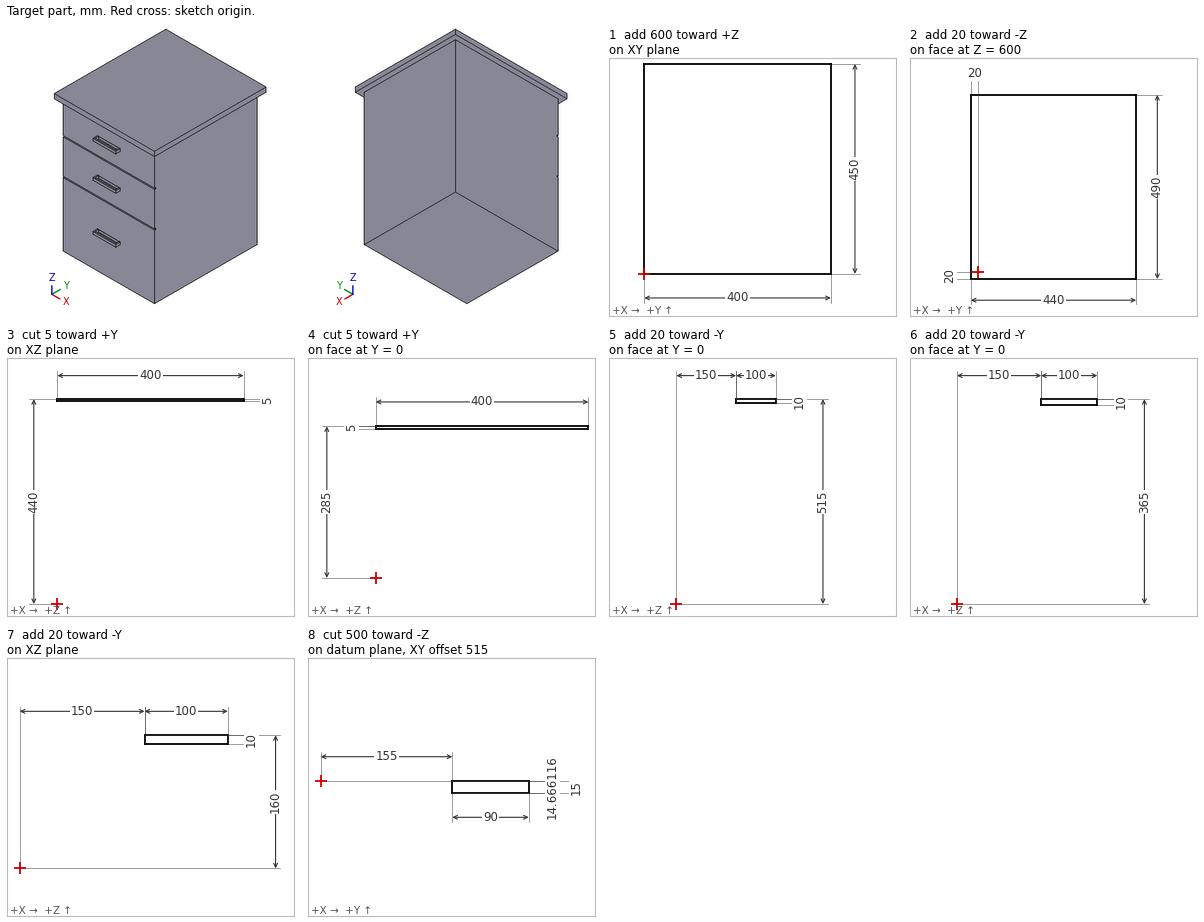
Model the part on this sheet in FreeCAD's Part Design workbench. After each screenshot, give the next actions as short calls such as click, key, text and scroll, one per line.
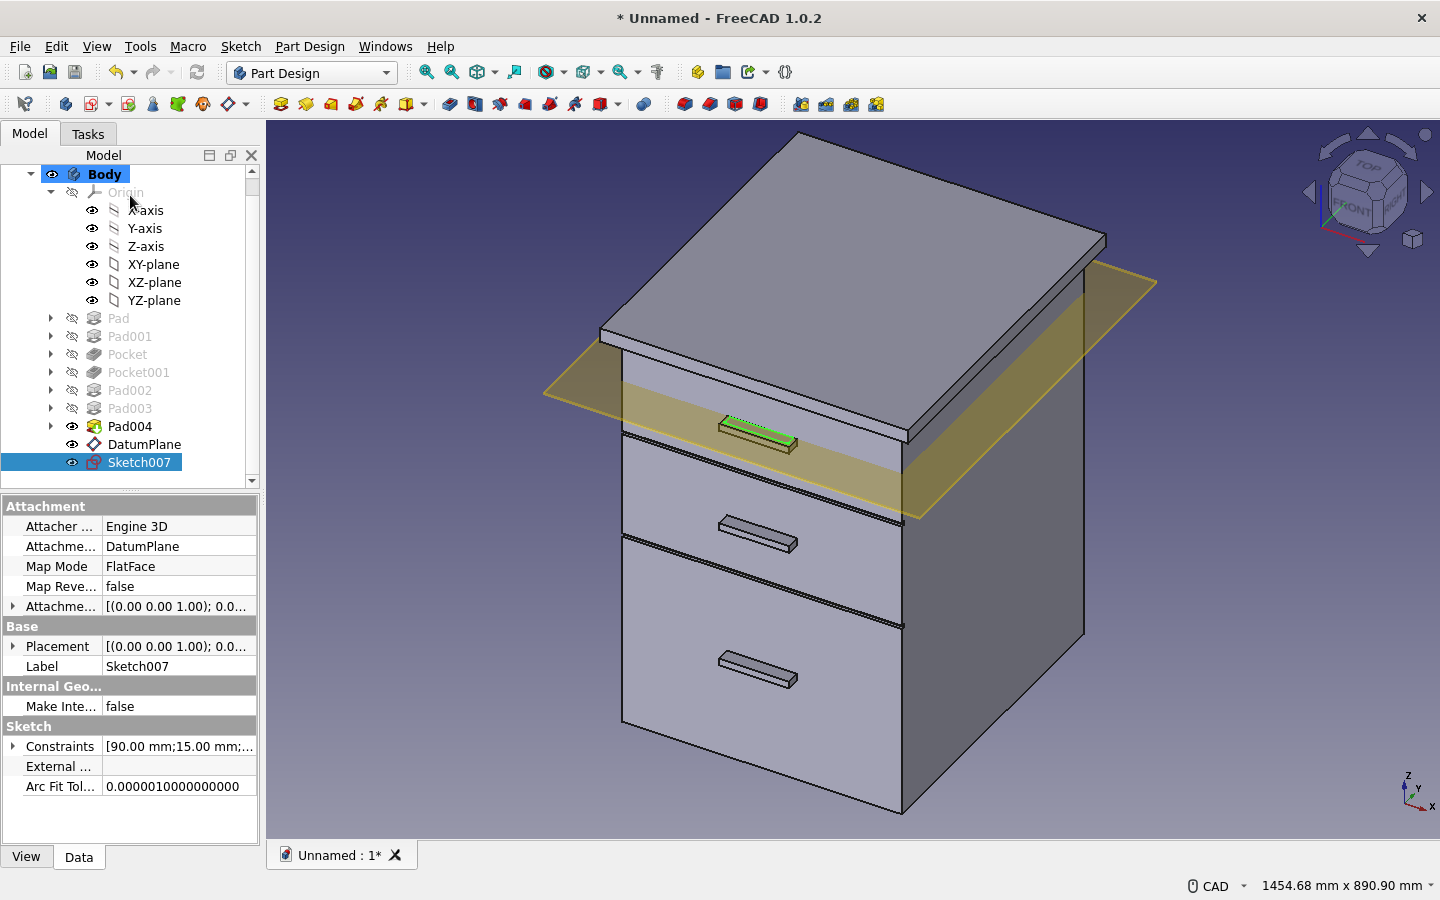
click(450, 104)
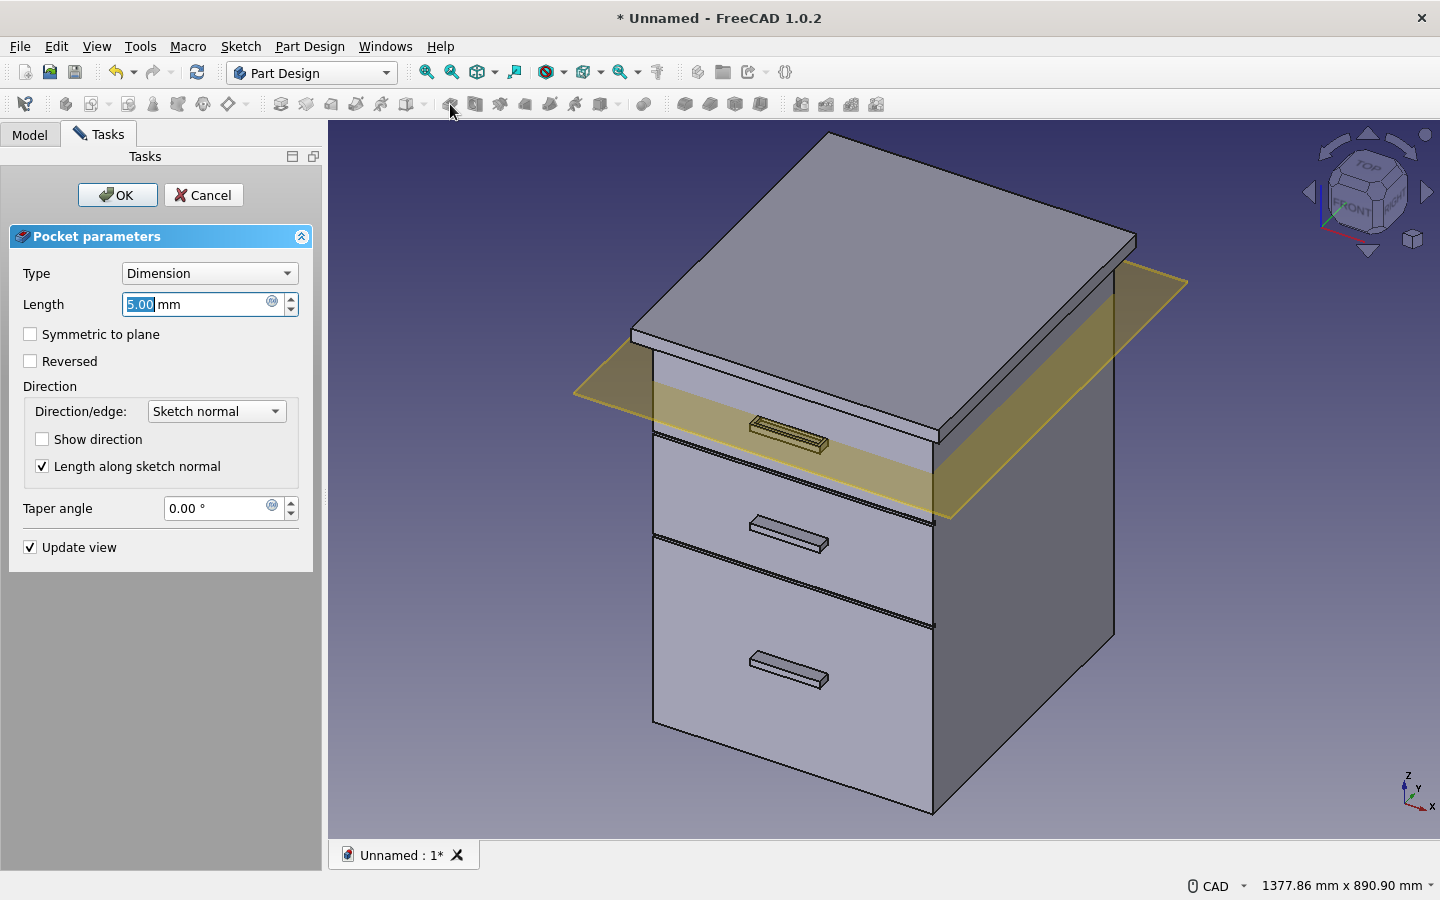
text(500)
key(Tab)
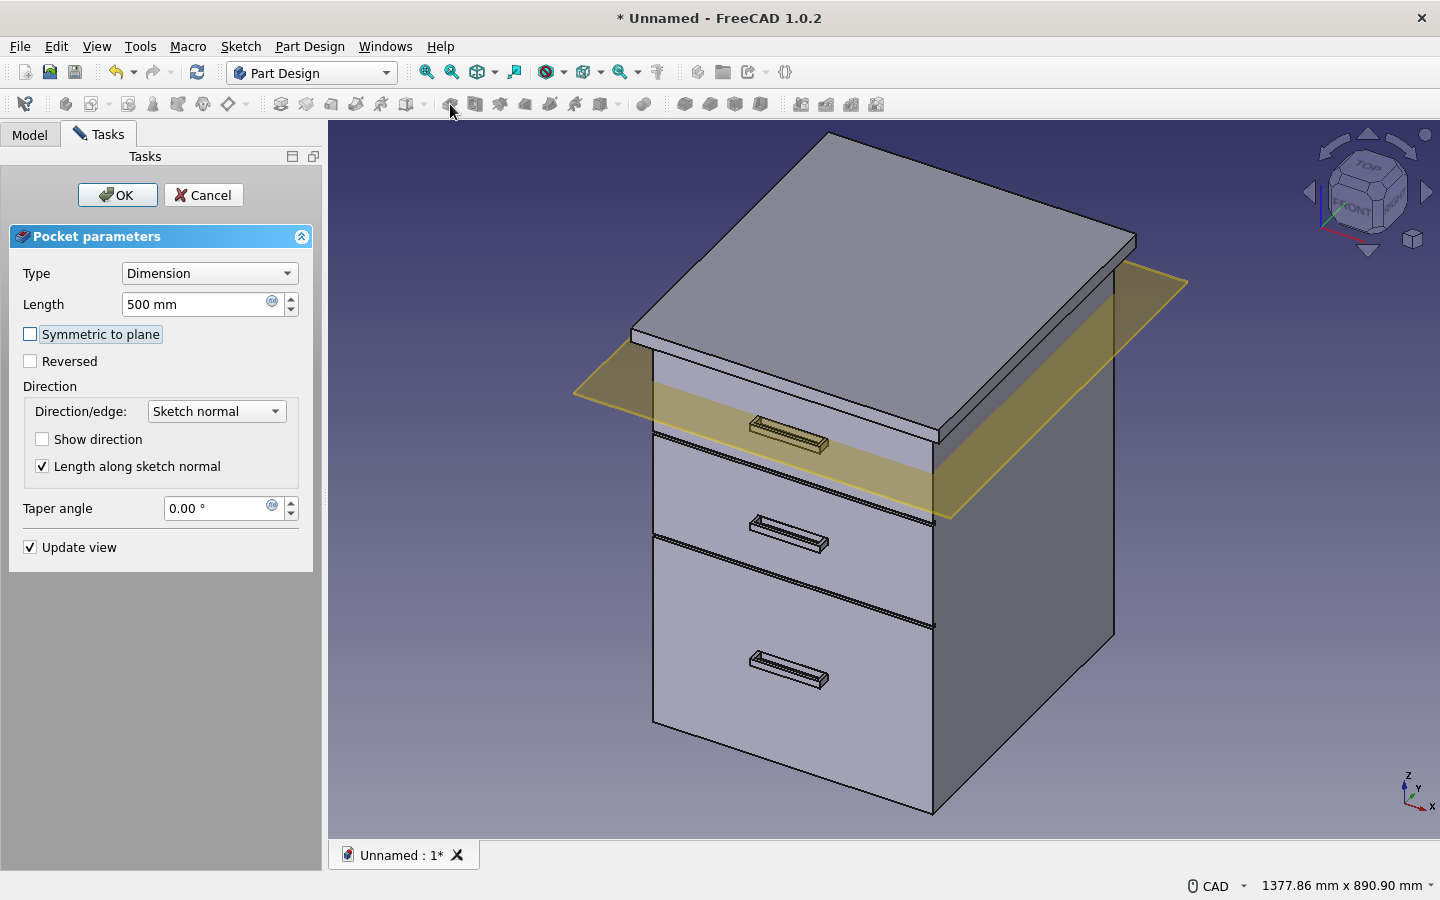
click(118, 195)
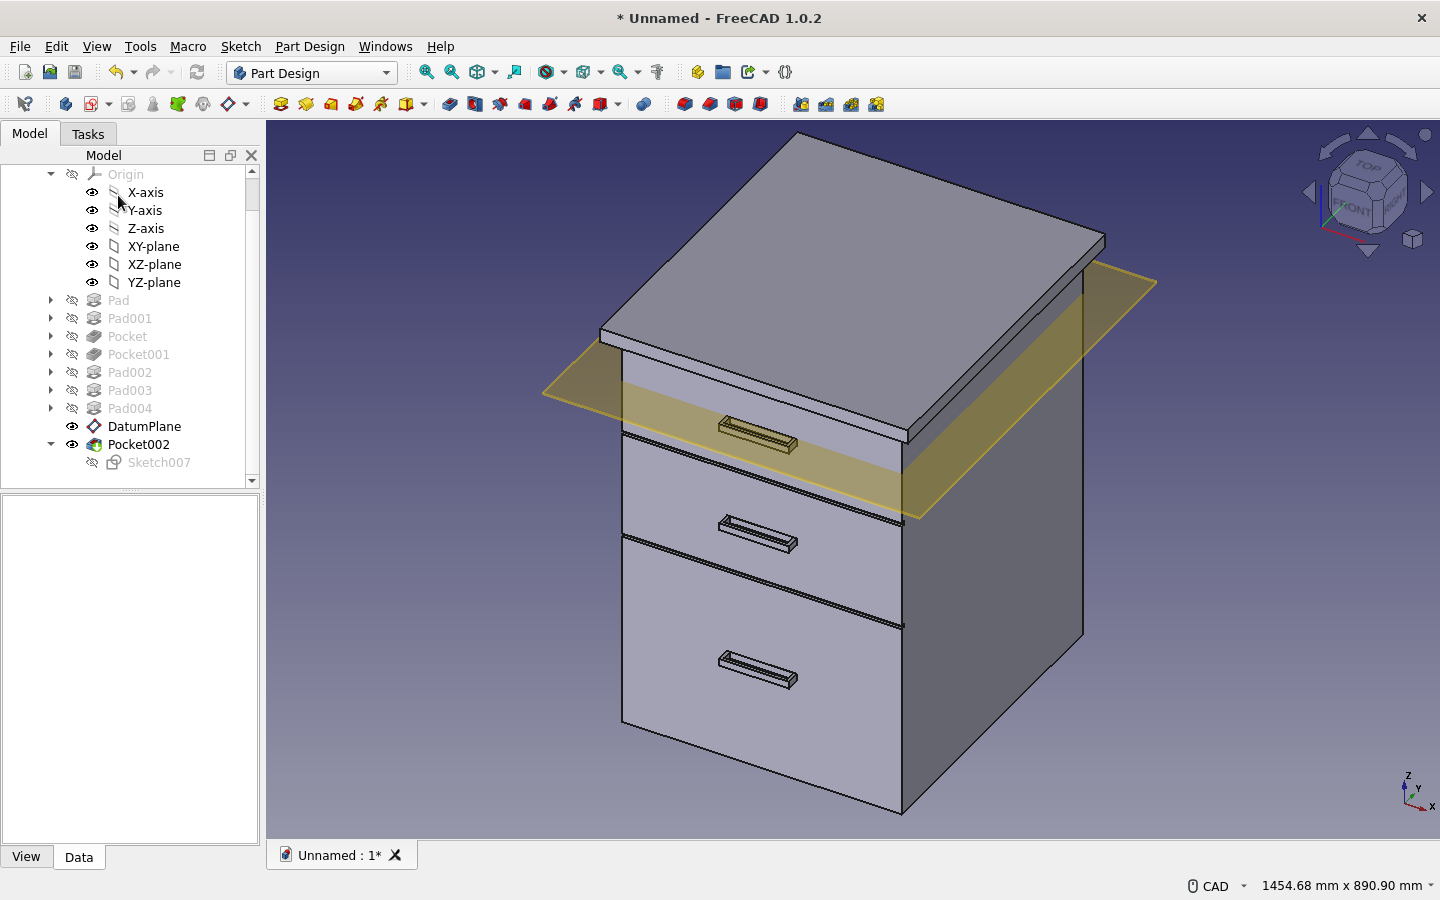
click(117, 426)
key(space)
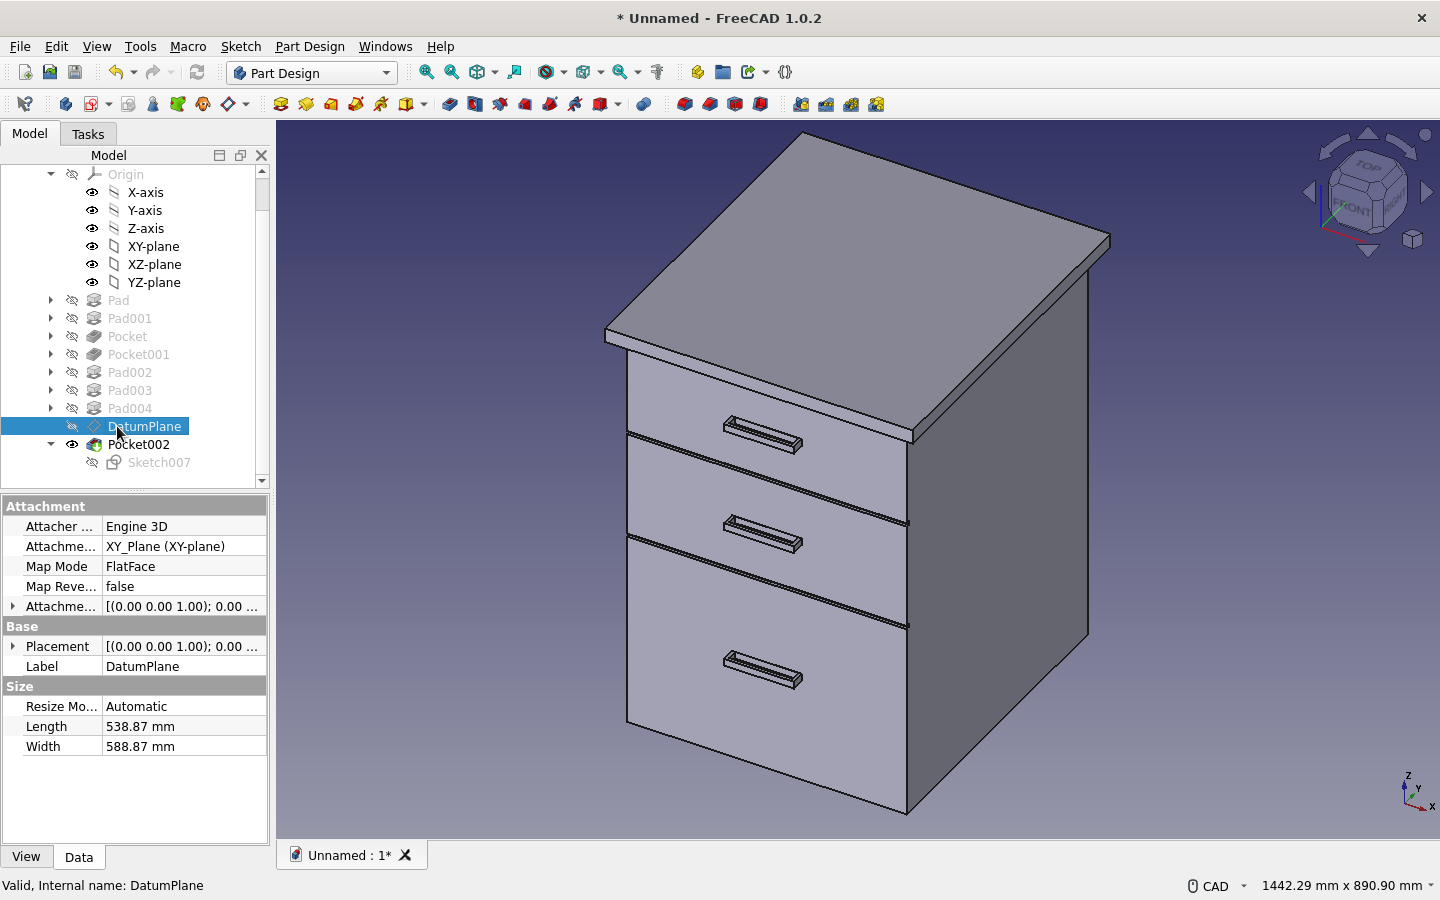
key(0)